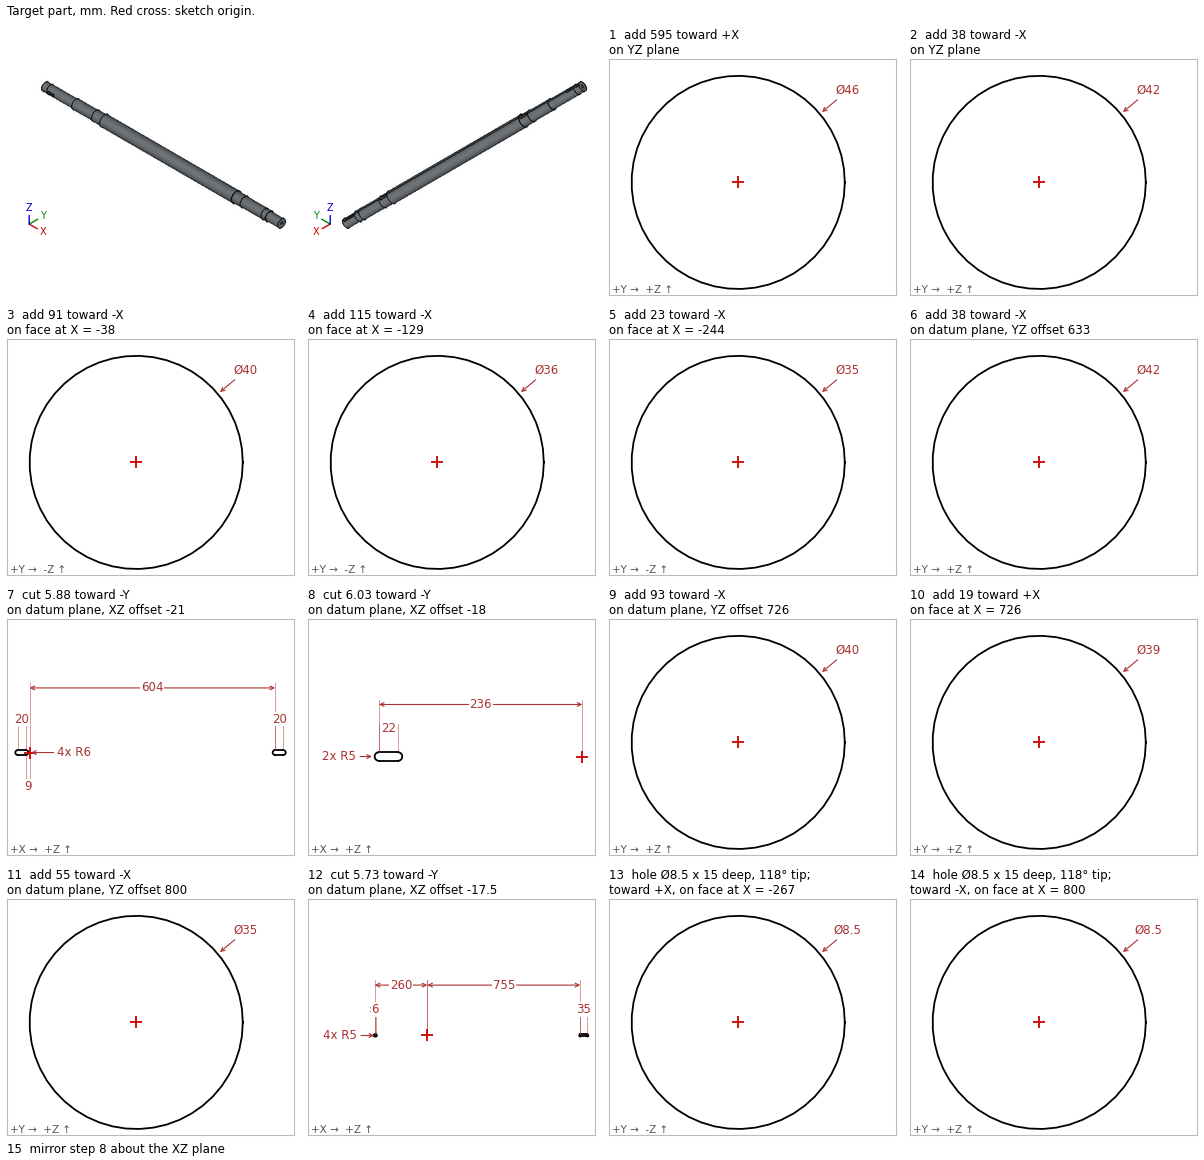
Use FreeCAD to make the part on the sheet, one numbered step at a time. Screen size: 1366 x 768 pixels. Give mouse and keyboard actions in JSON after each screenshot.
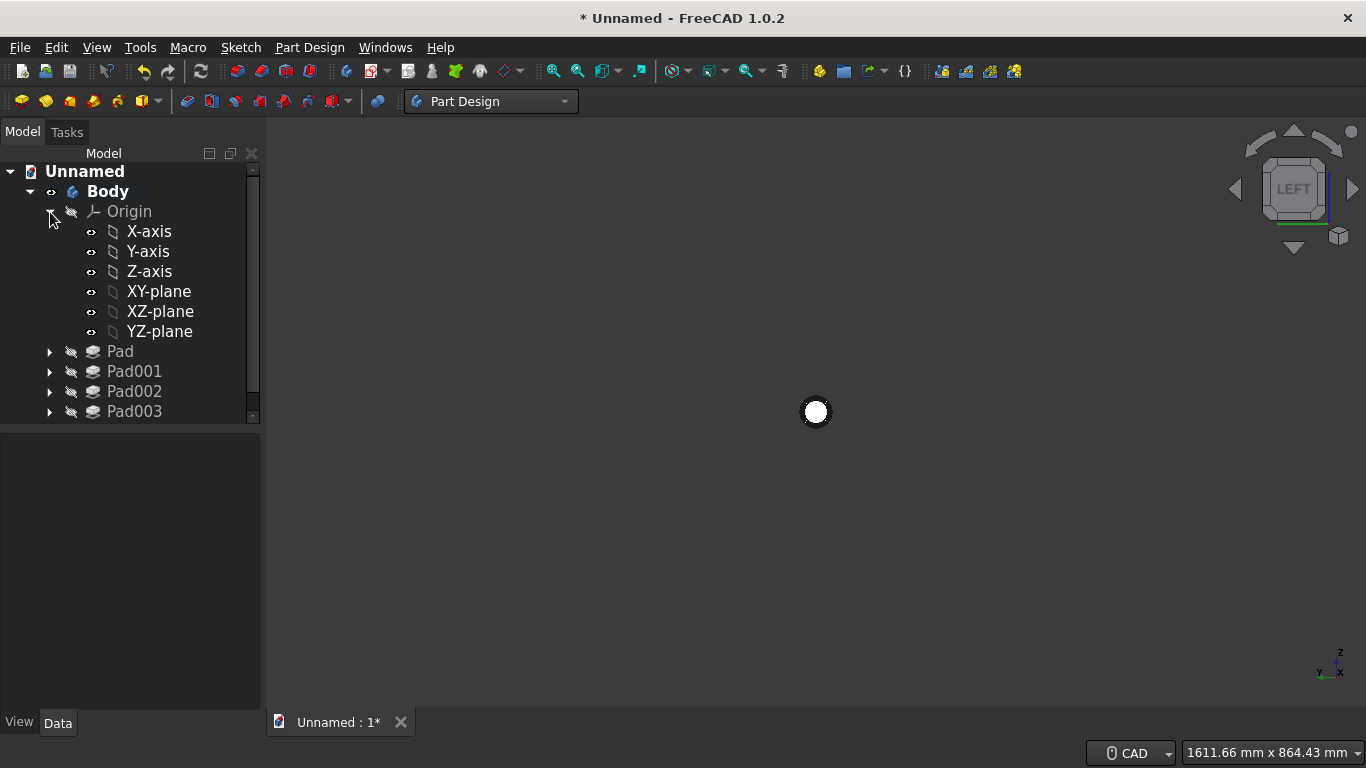
{"action": "left_click", "coordinate": [136, 332]}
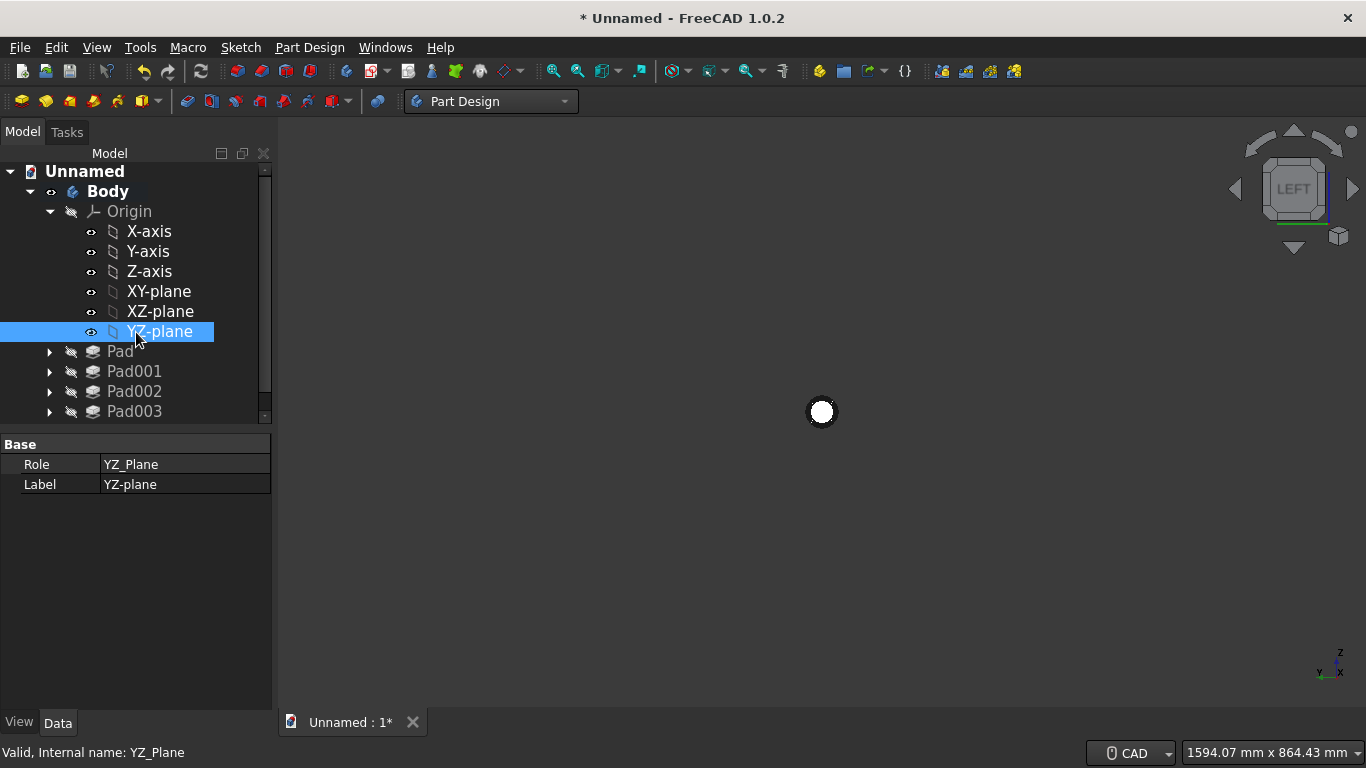
{"action": "left_click", "coordinate": [504, 72]}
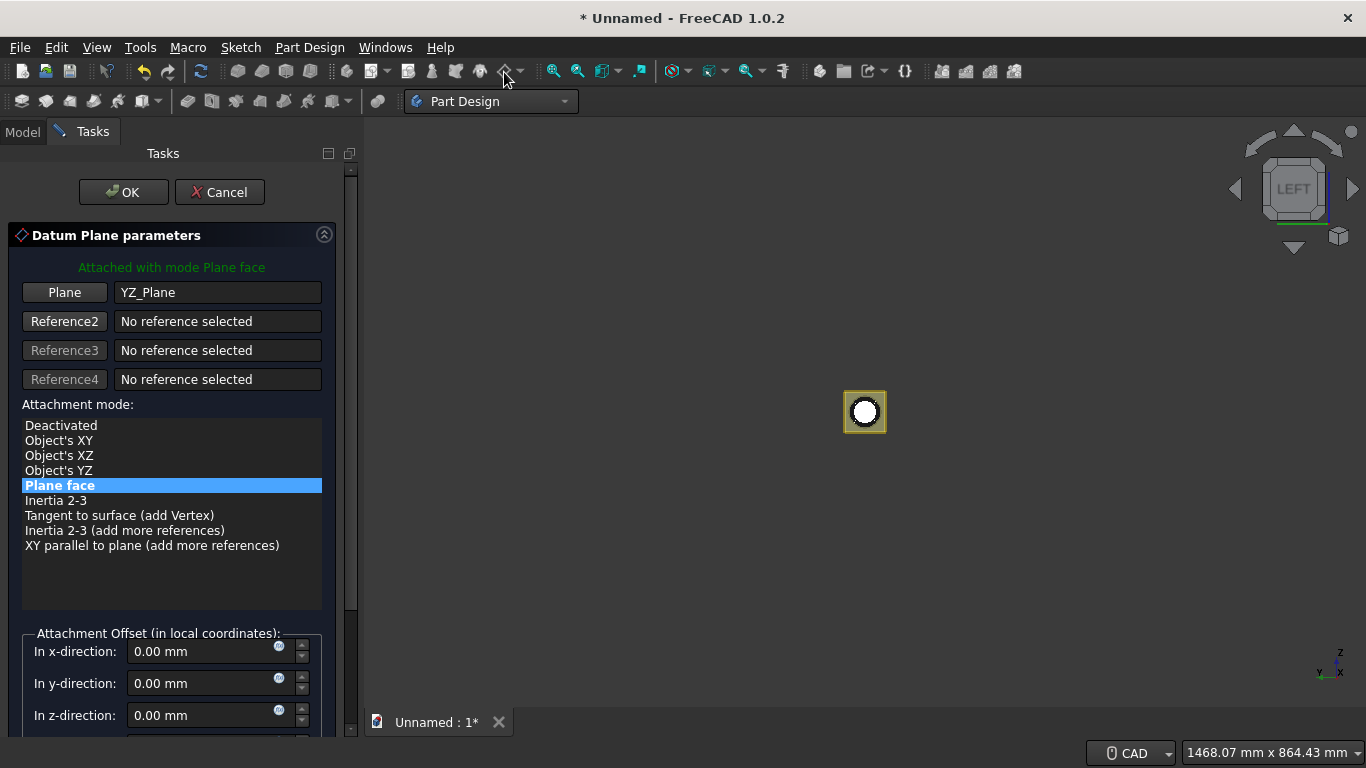
{"action": "triple_click", "coordinate": [210, 715]}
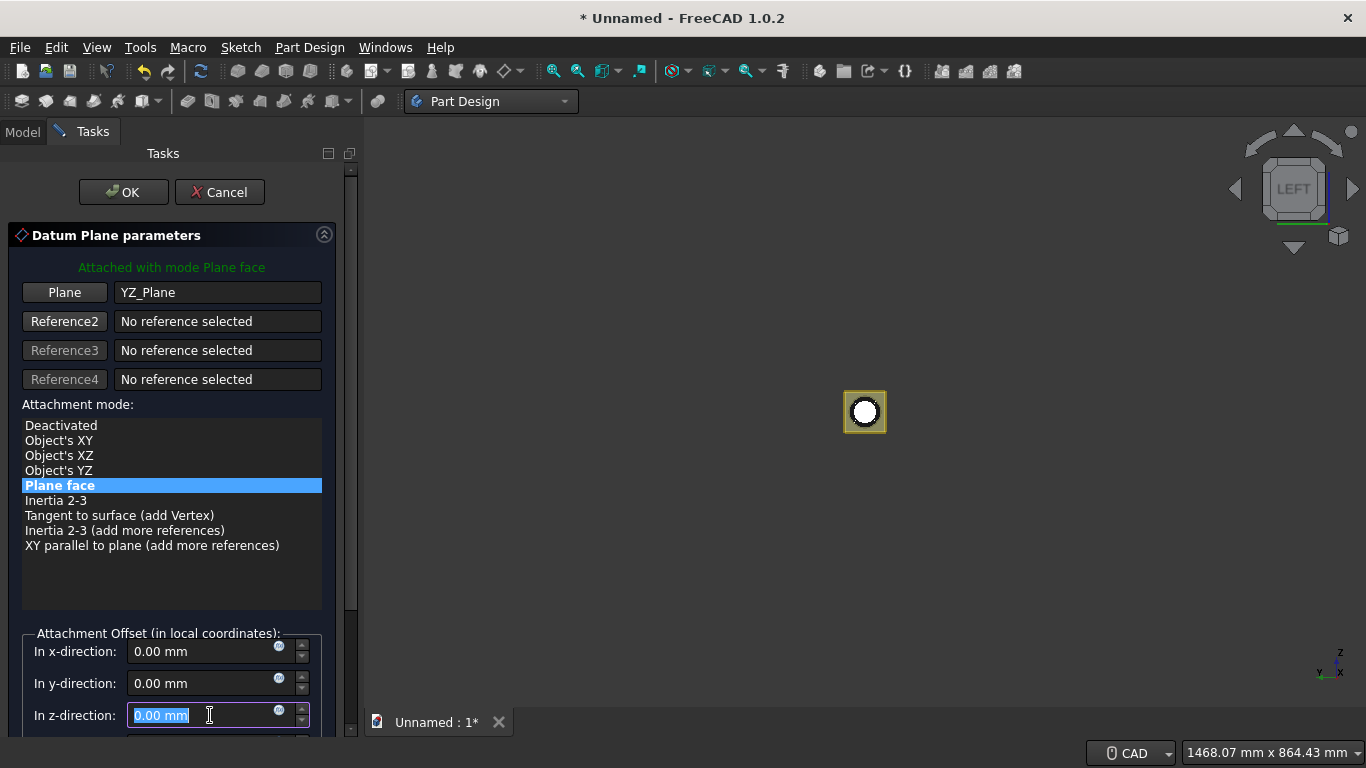
{"action": "type", "text": "633"}
{"action": "key", "text": "Tab"}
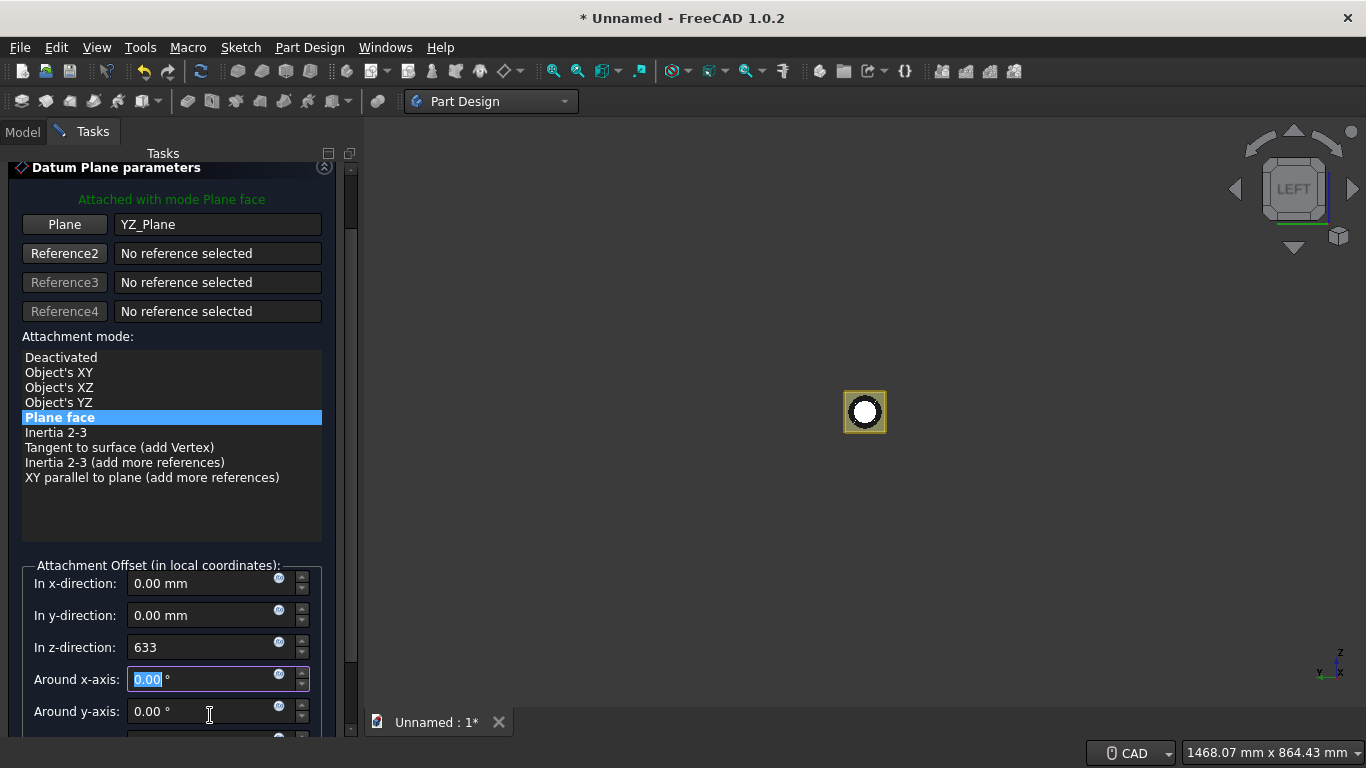
{"action": "scroll", "coordinate": [351, 450], "scroll_direction": "up", "scroll_amount": 2}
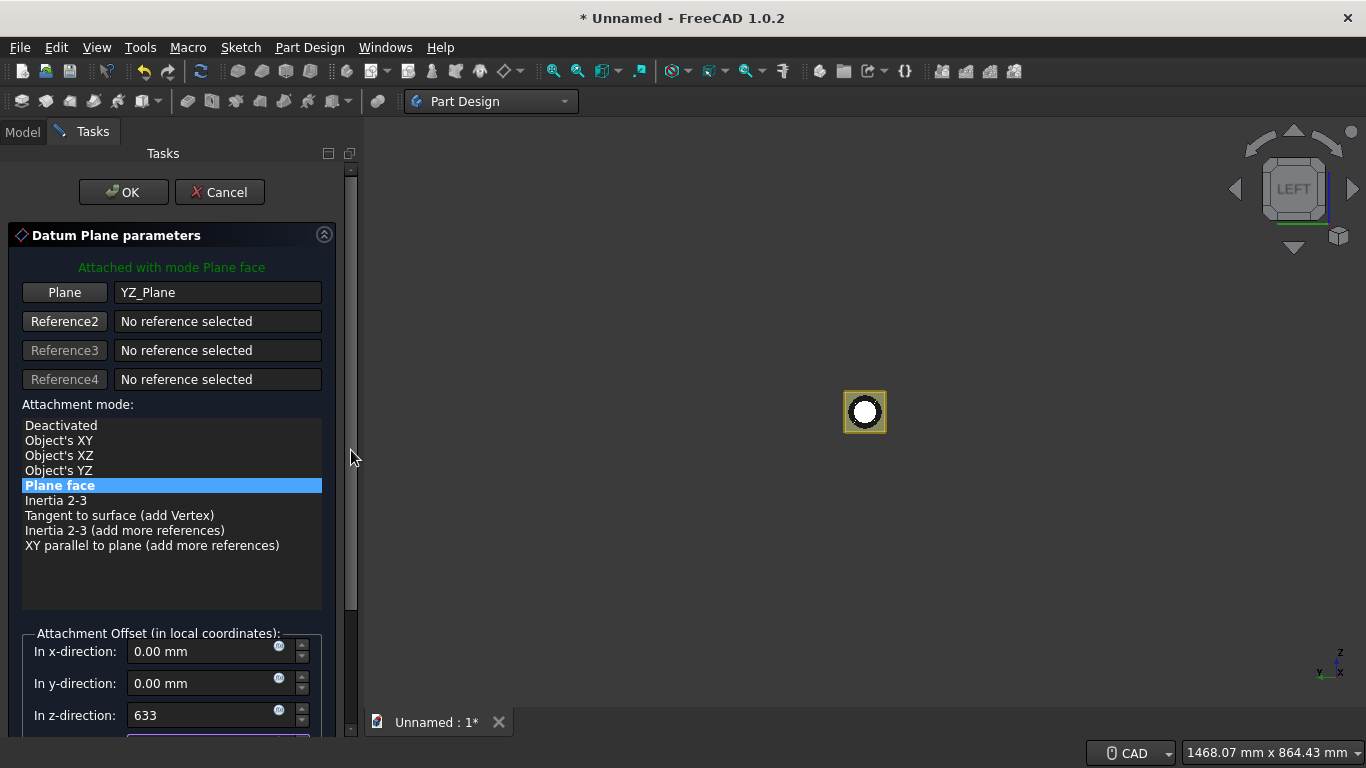
{"action": "left_click", "coordinate": [124, 192]}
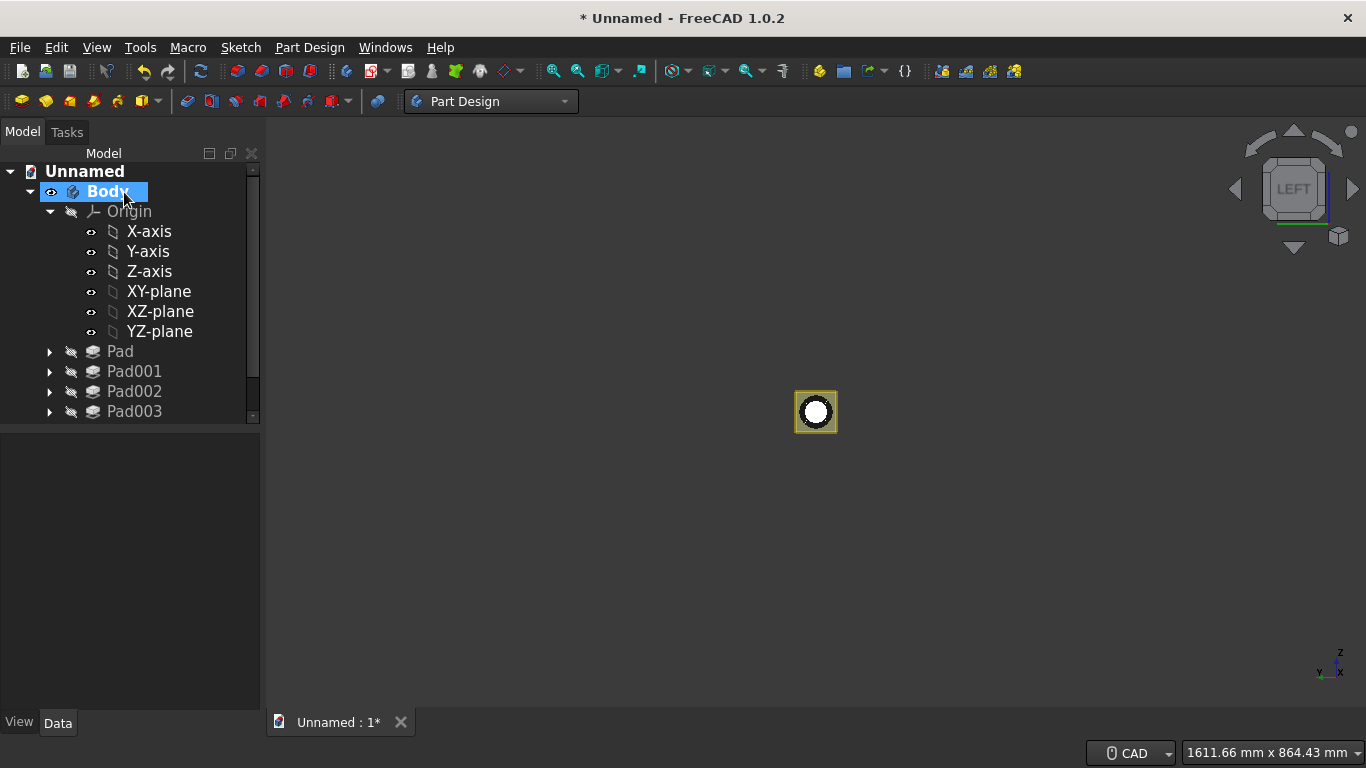
{"action": "scroll", "coordinate": [100, 287], "scroll_direction": "down", "scroll_amount": 3}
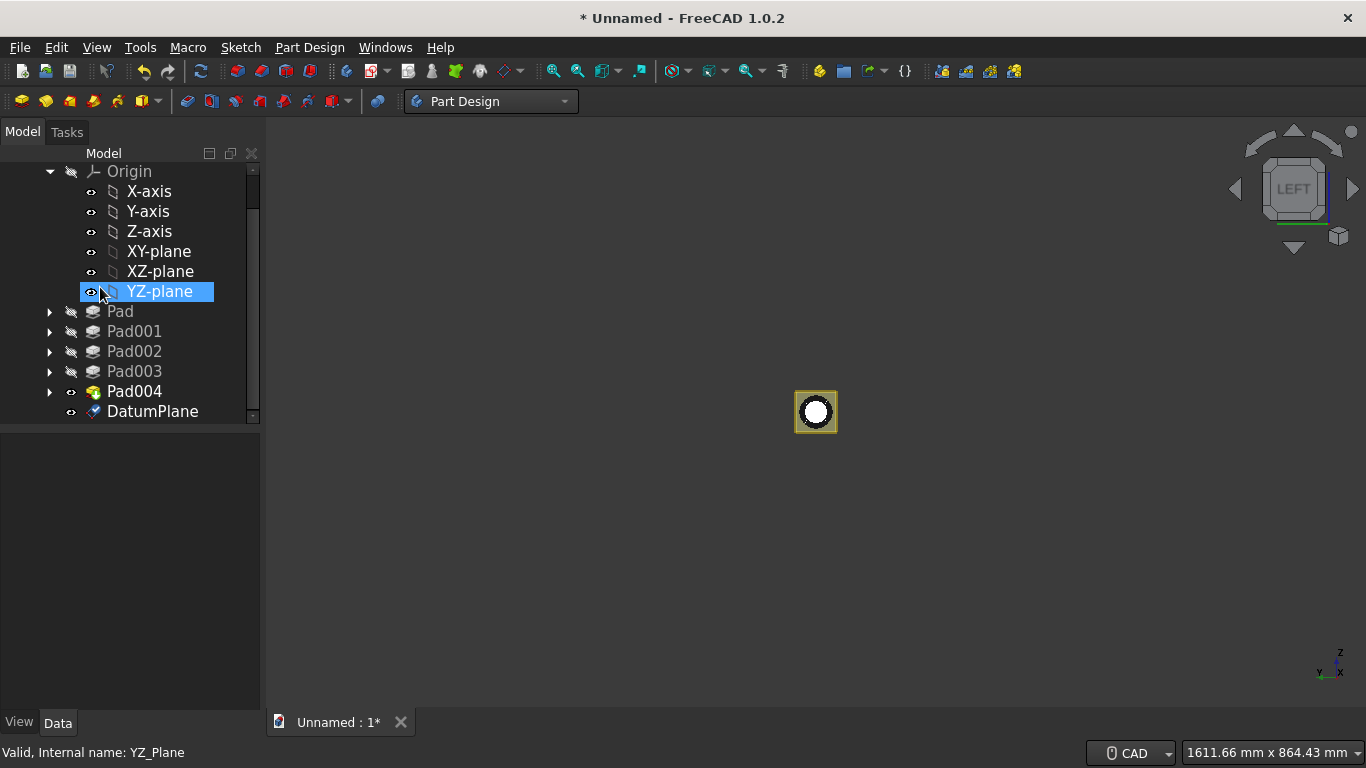
{"action": "left_click", "coordinate": [116, 412]}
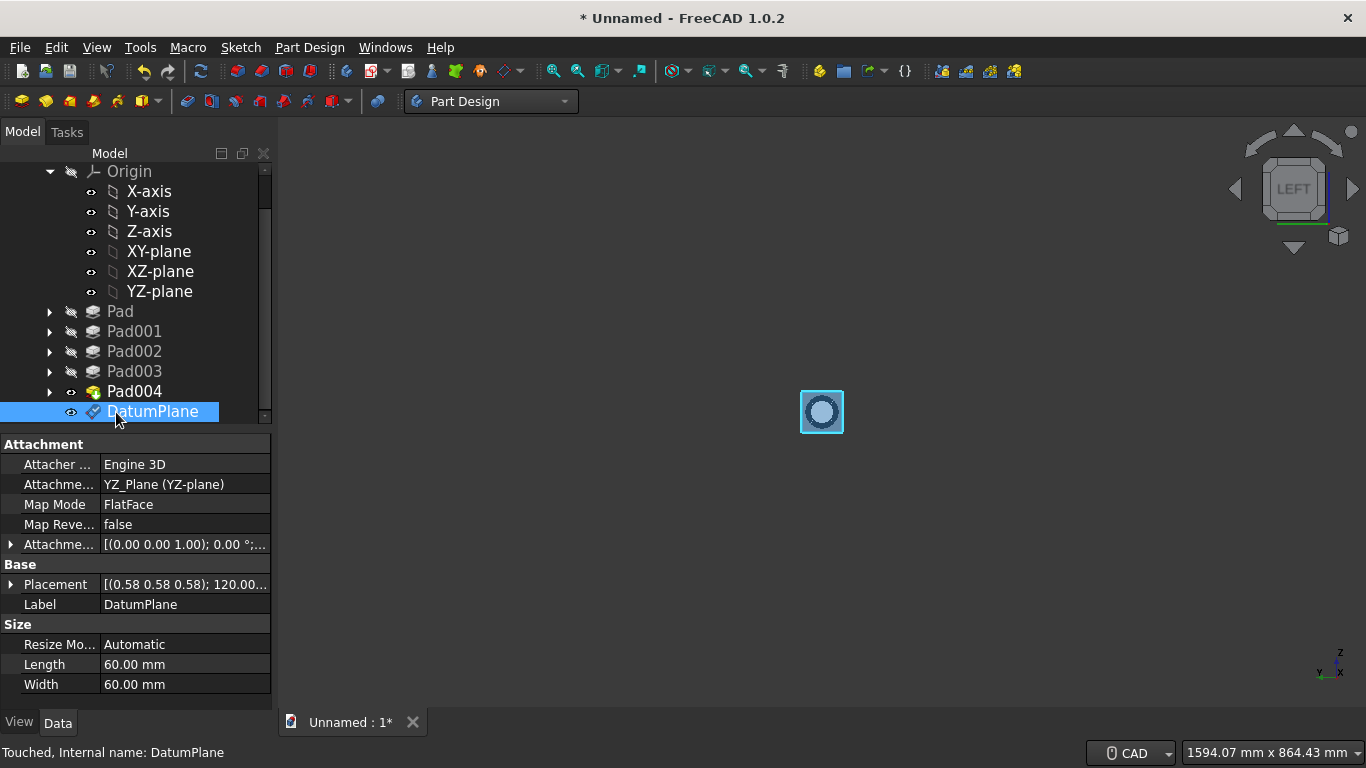
{"action": "left_click", "coordinate": [372, 72]}